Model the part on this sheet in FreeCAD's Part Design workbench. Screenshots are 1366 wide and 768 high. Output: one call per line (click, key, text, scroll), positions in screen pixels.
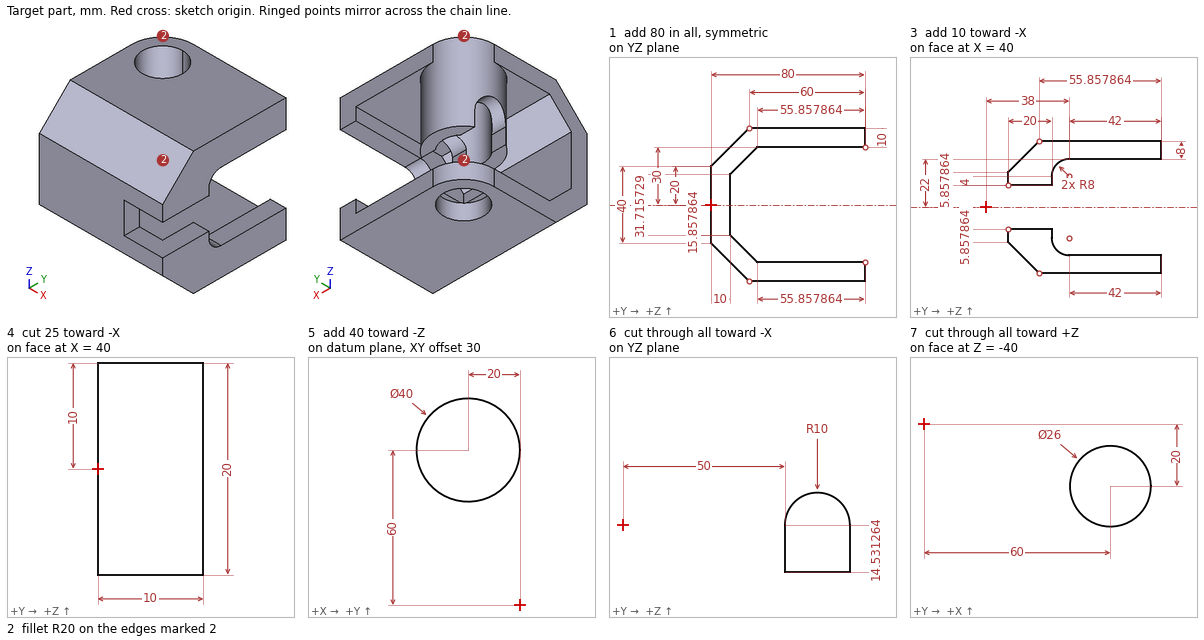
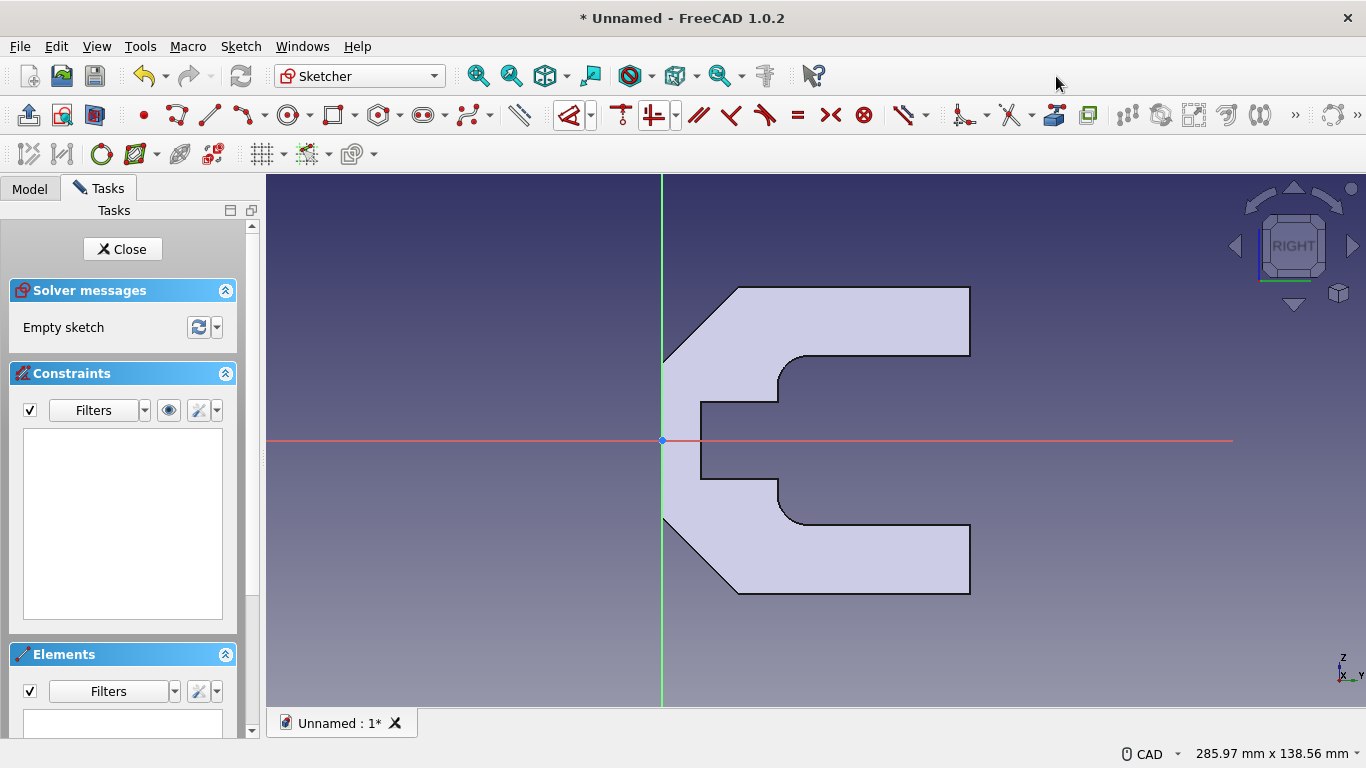
scroll(660, 440, up, 7)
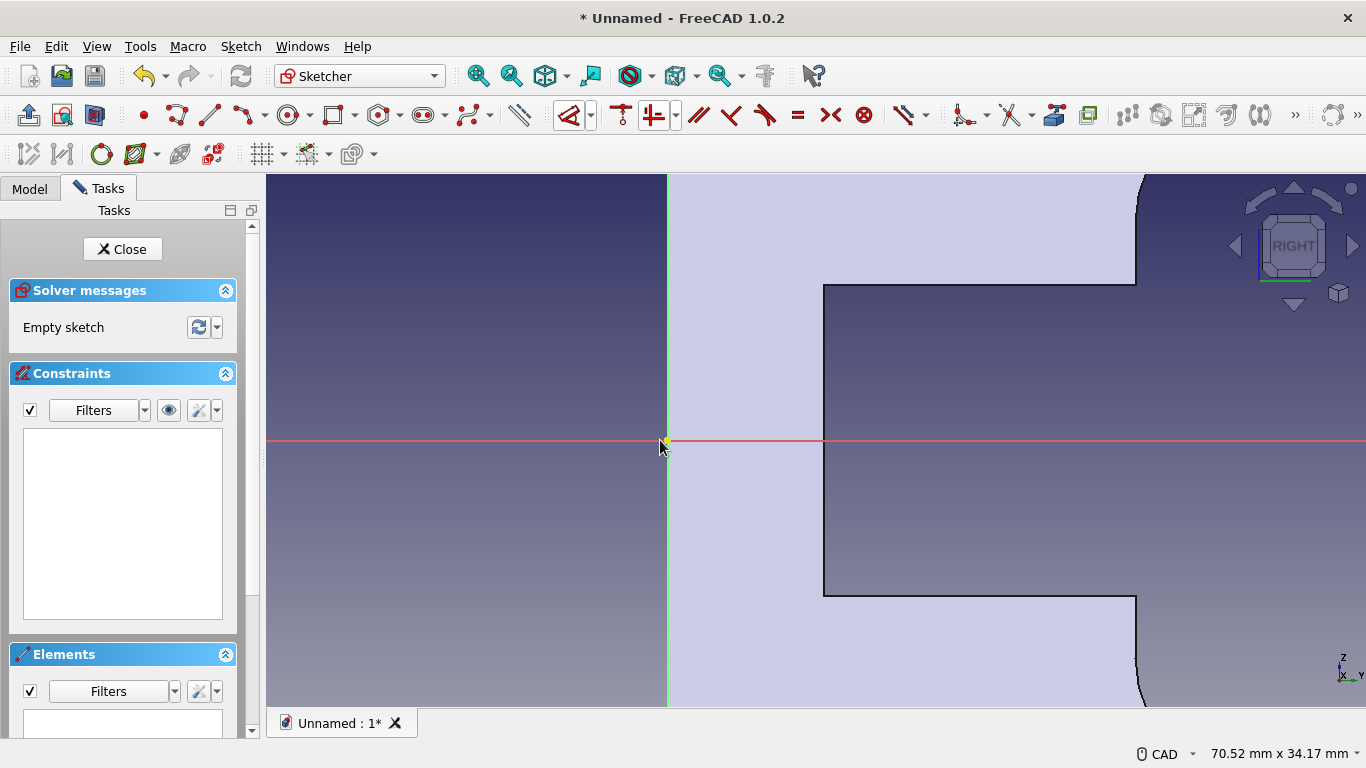
click(332, 116)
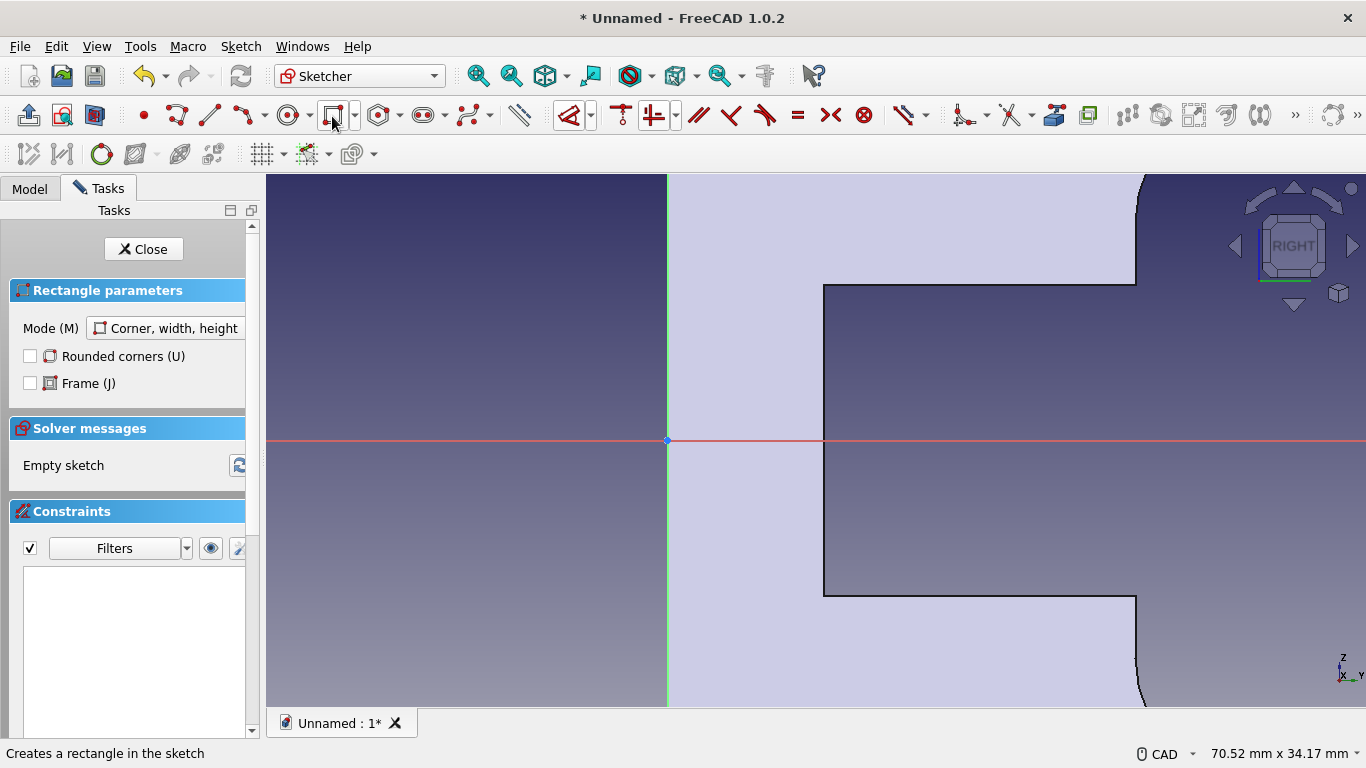
click(668, 285)
move(824, 596)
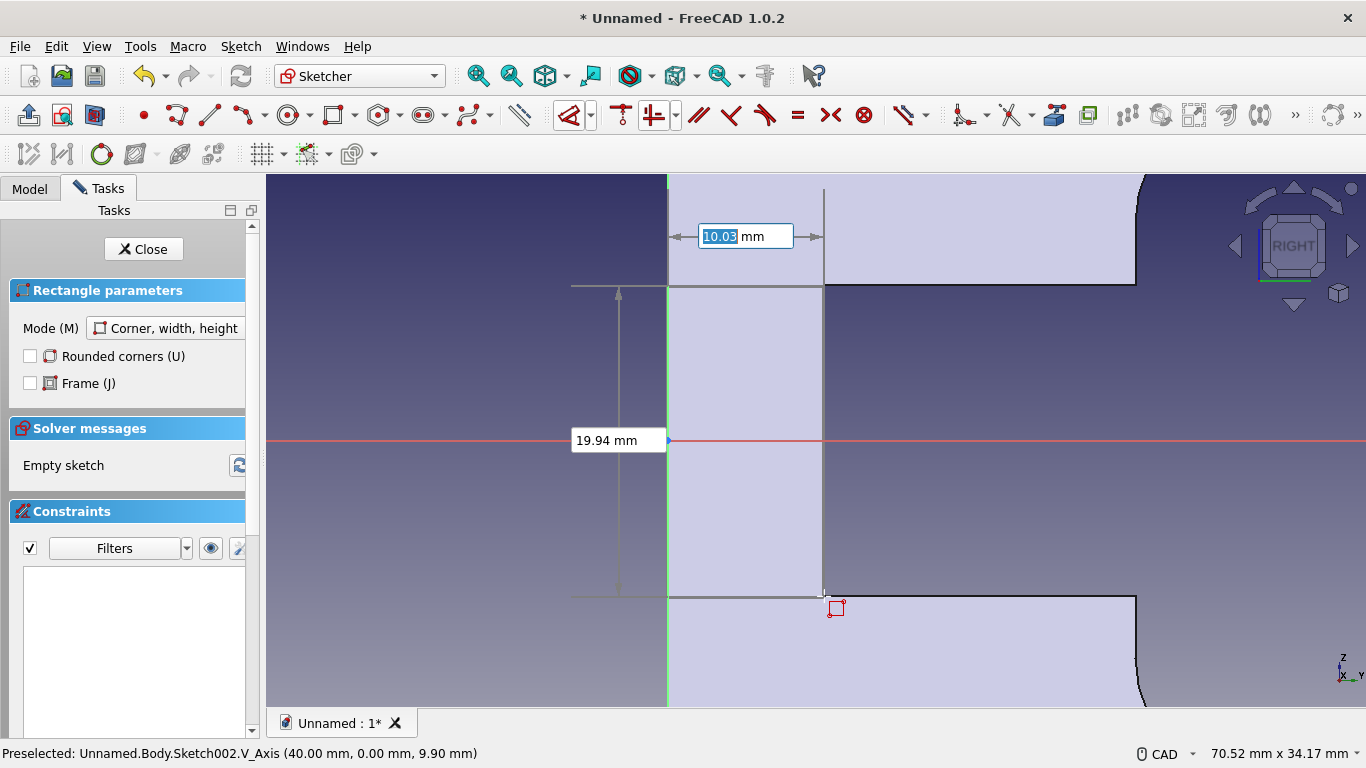
text(10)
key(Tab)
text(20)
key(Return)
key(Escape)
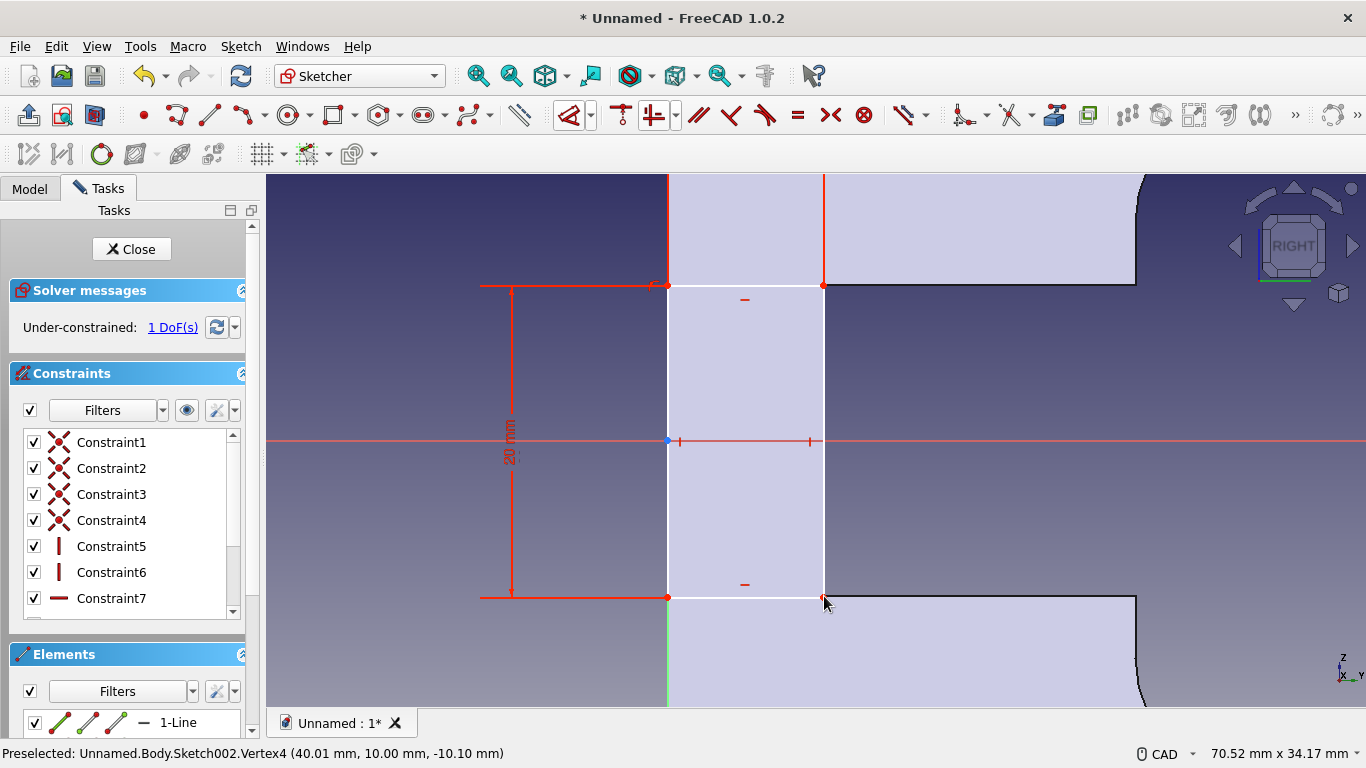
click(668, 286)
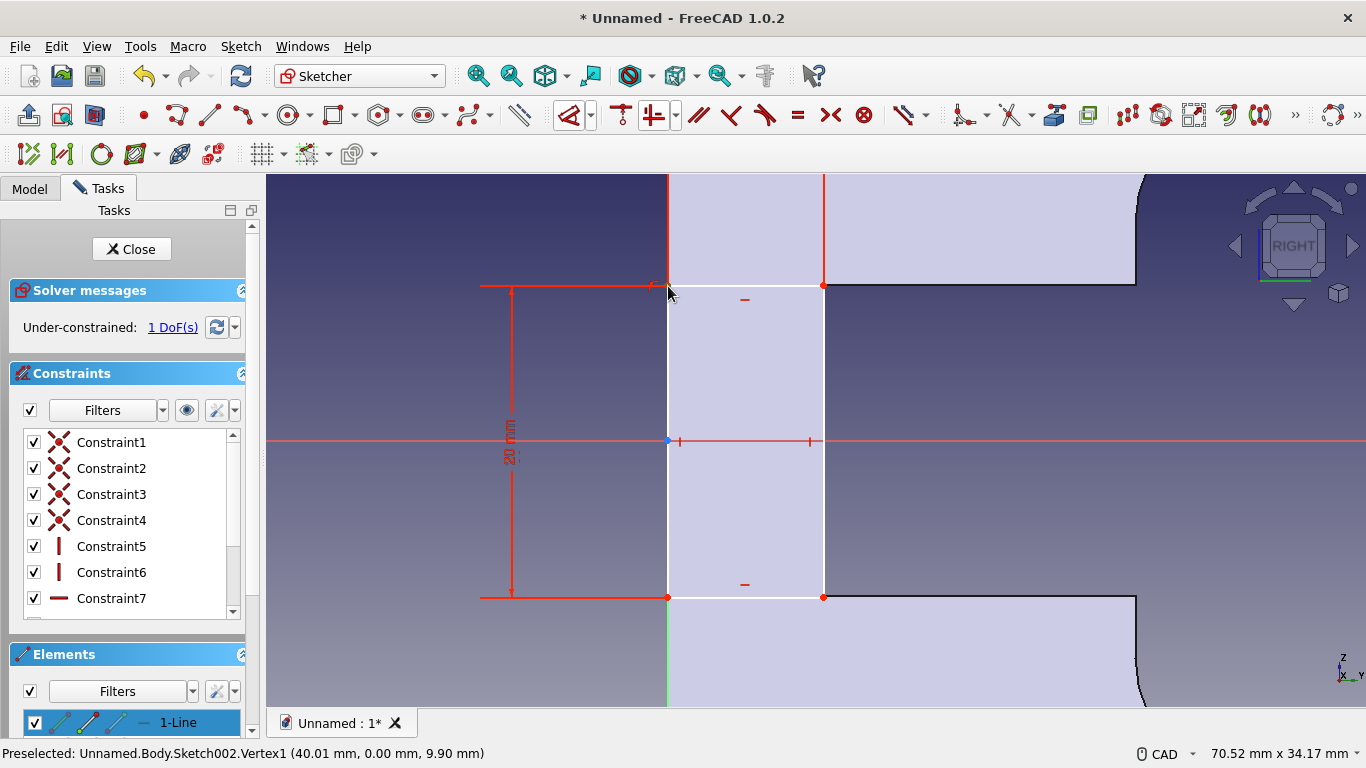
click(590, 116)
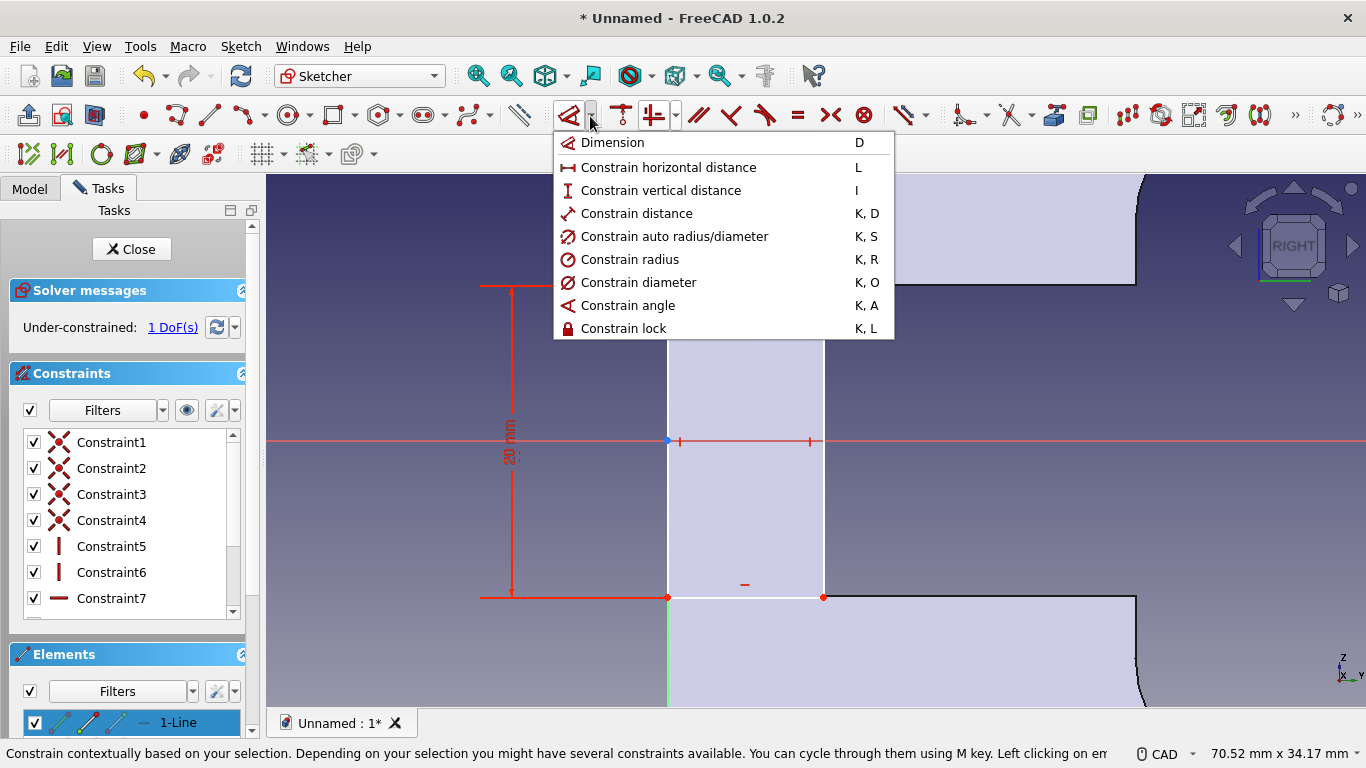
click(724, 190)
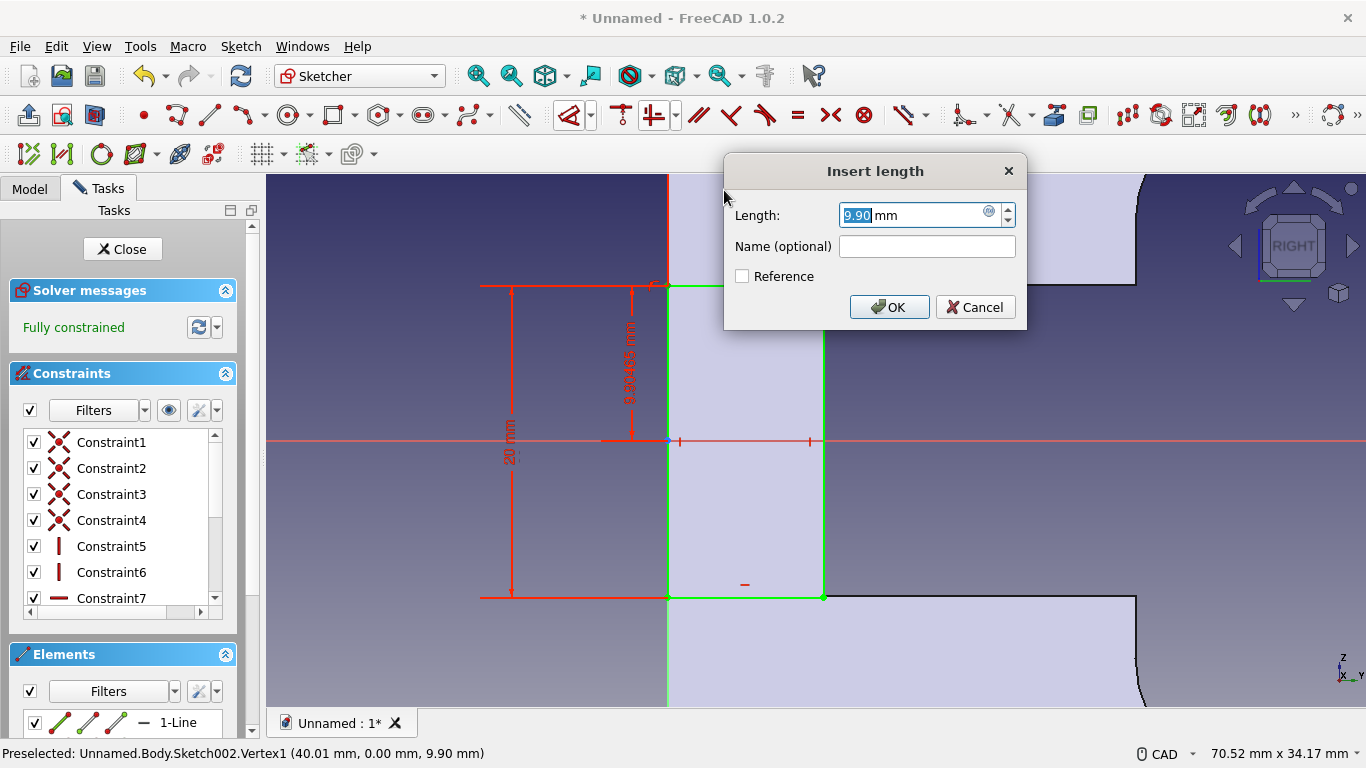
text(10)
key(Return)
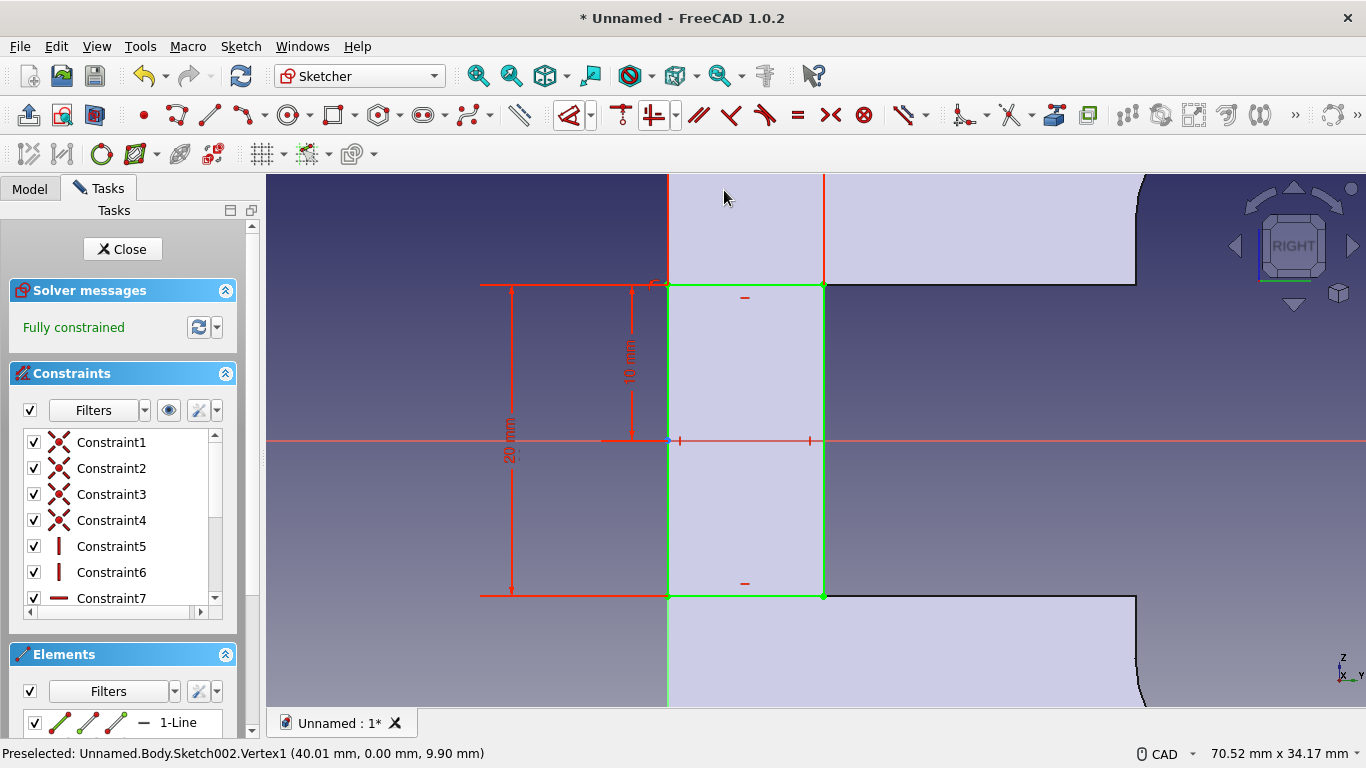
click(123, 249)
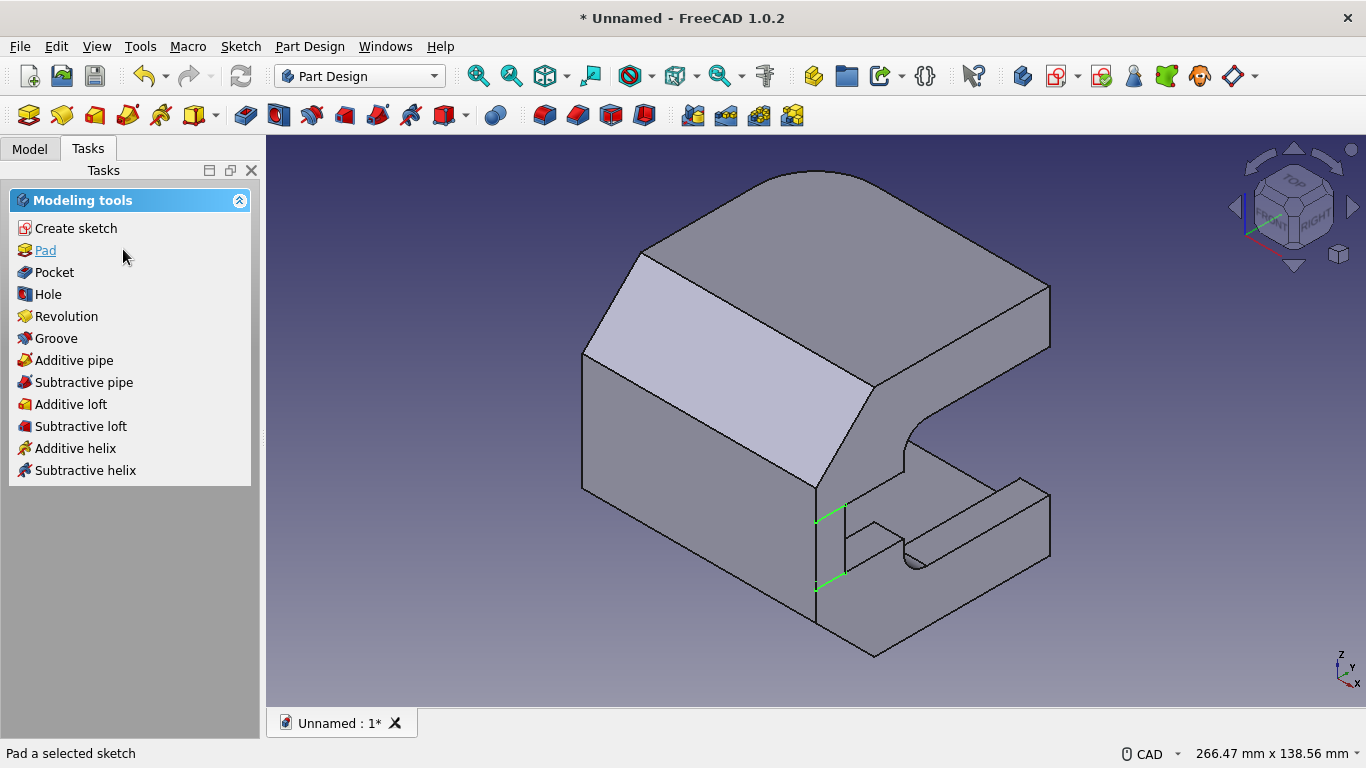
click(246, 116)